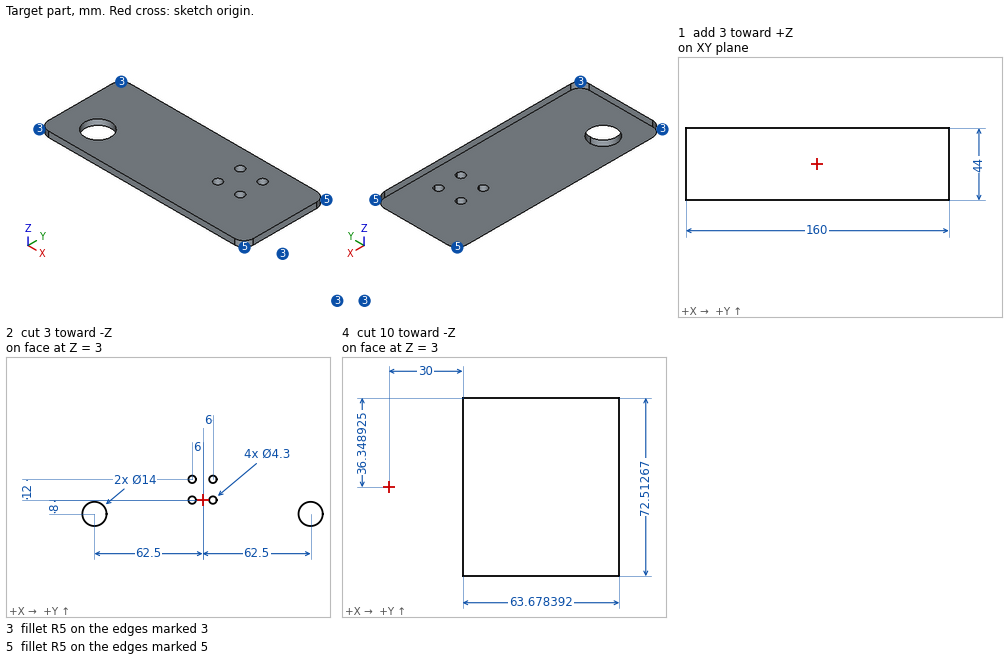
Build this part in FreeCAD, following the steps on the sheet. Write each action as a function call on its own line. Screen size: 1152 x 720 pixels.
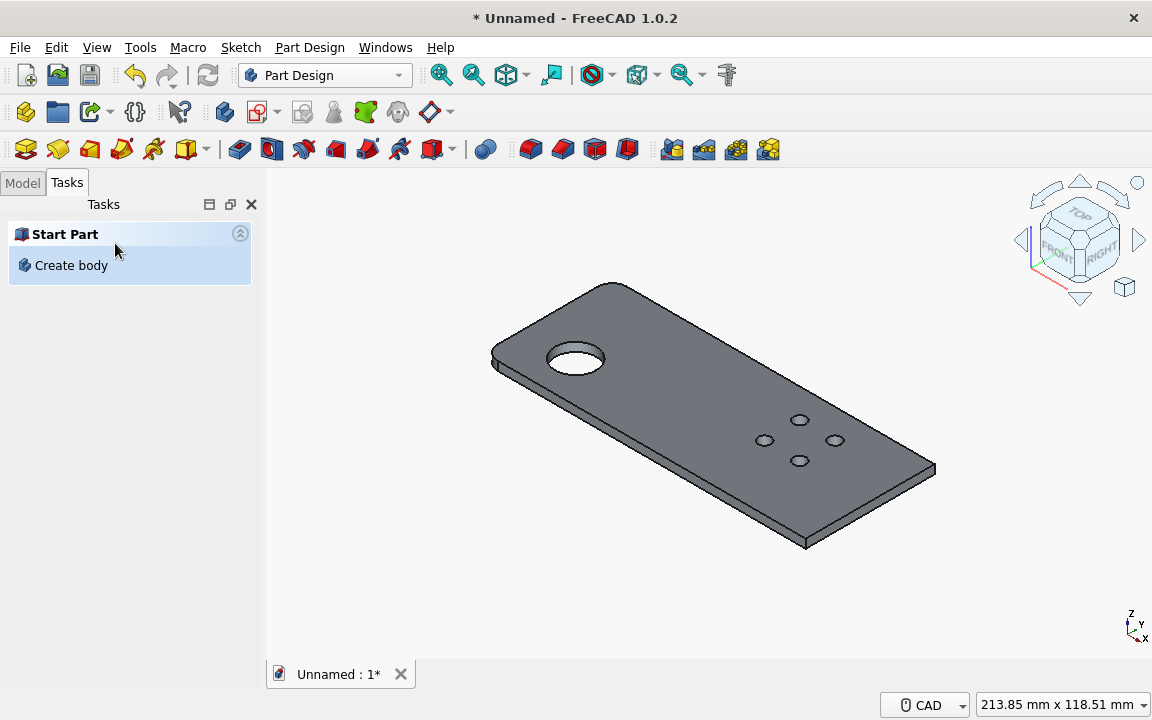
click(806, 544)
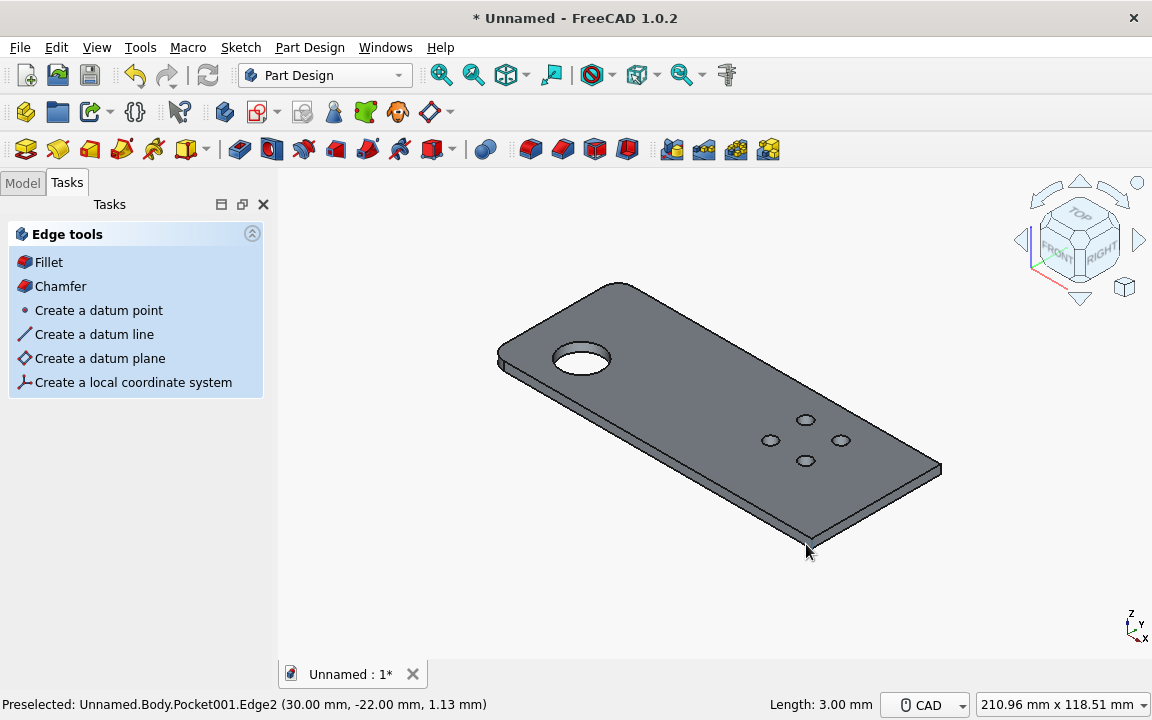
scroll(941, 468, up, 6)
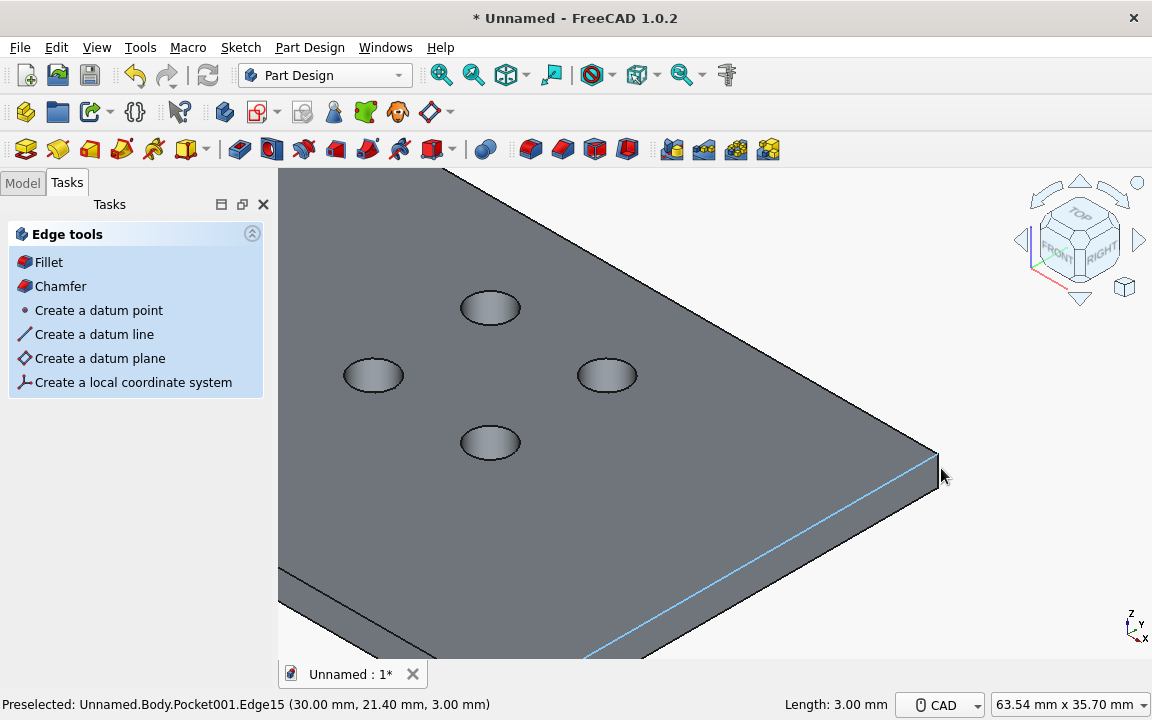
key(v)
key(f)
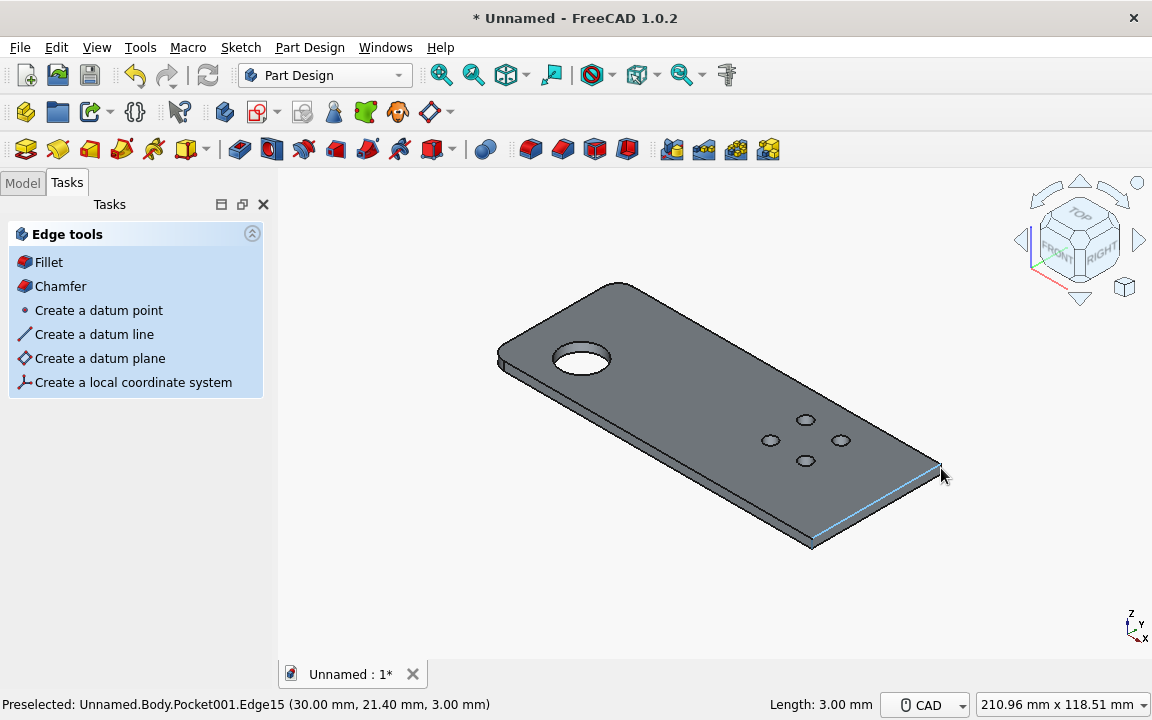
key(2)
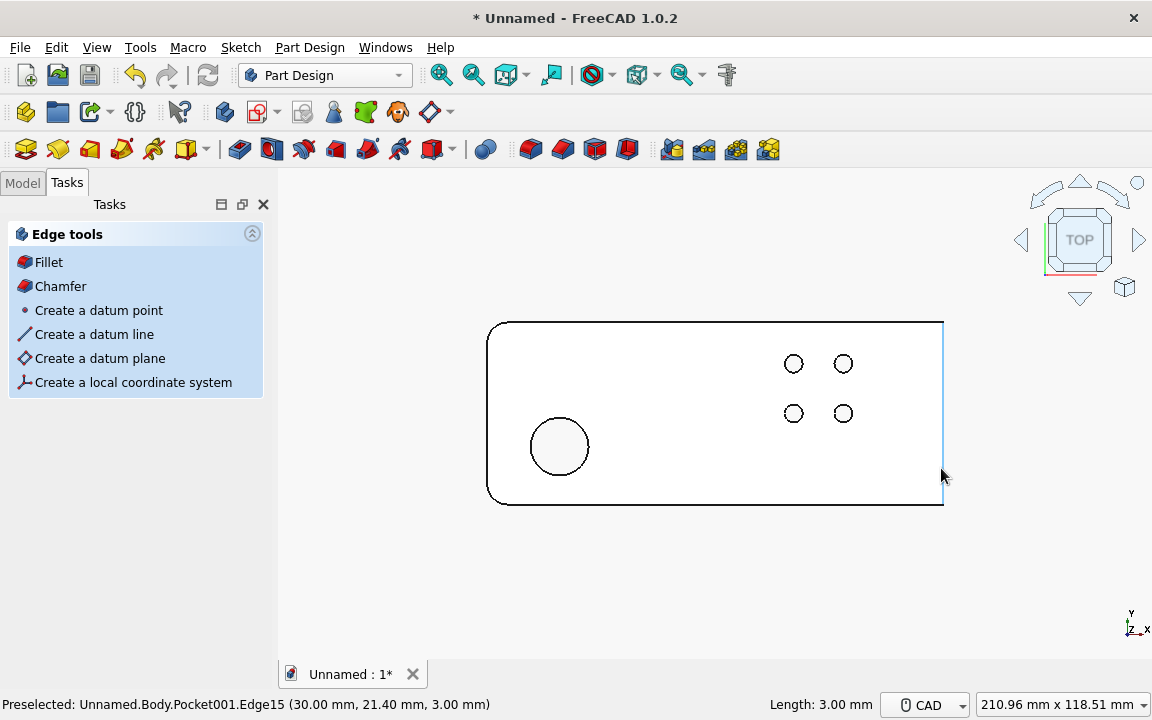
scroll(943, 321, up, 6)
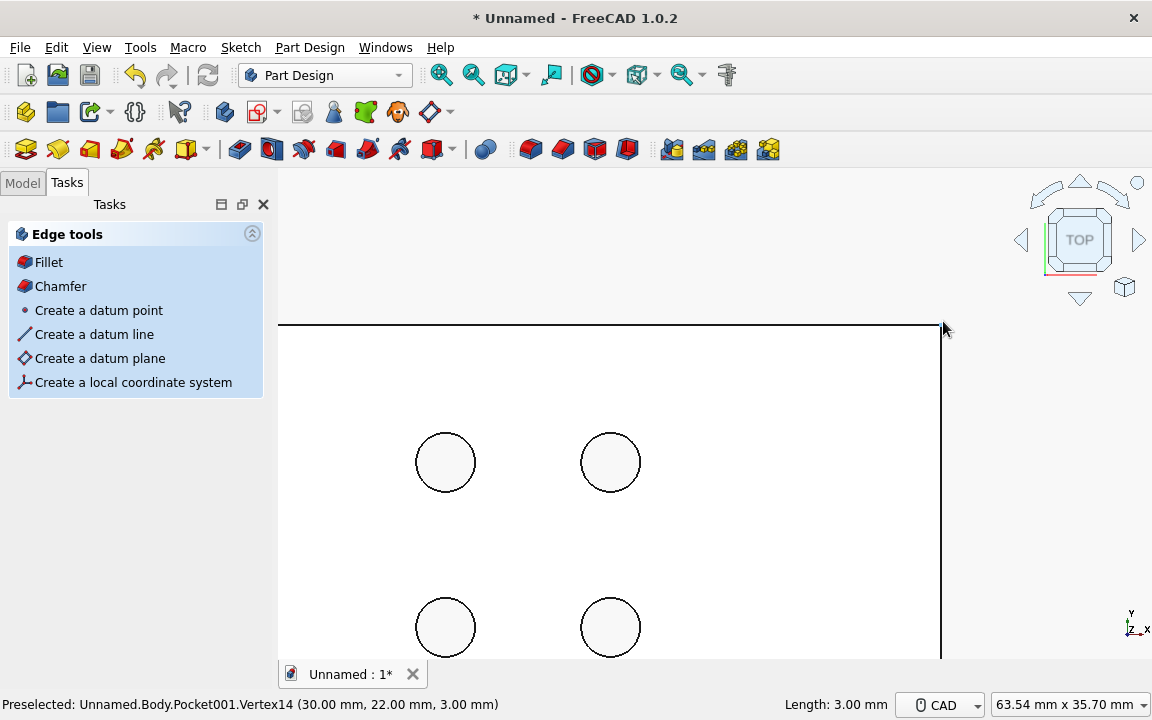
key(v)
key(f)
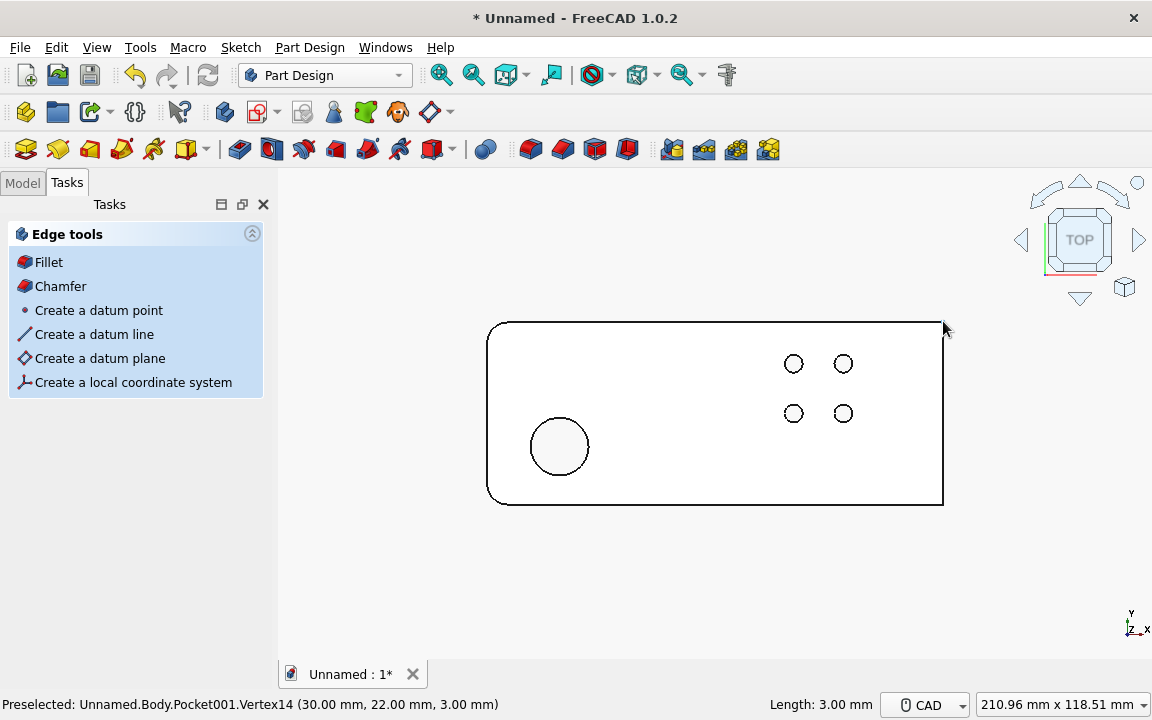
key(0)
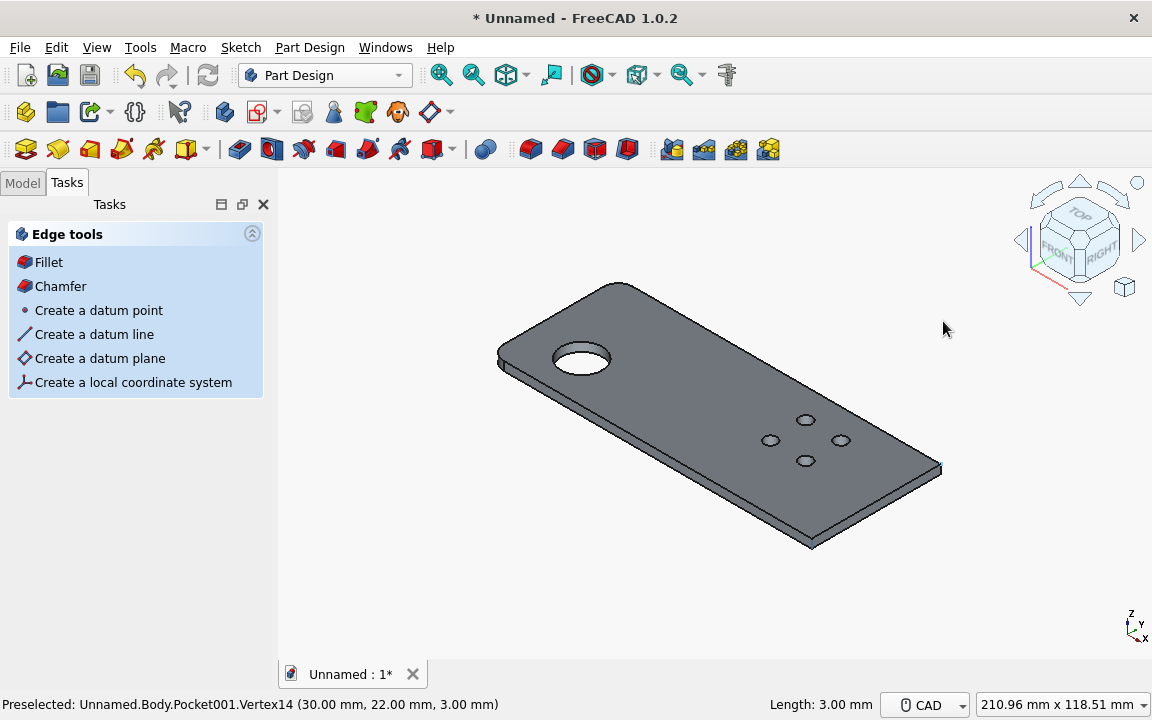
scroll(941, 468, up, 6)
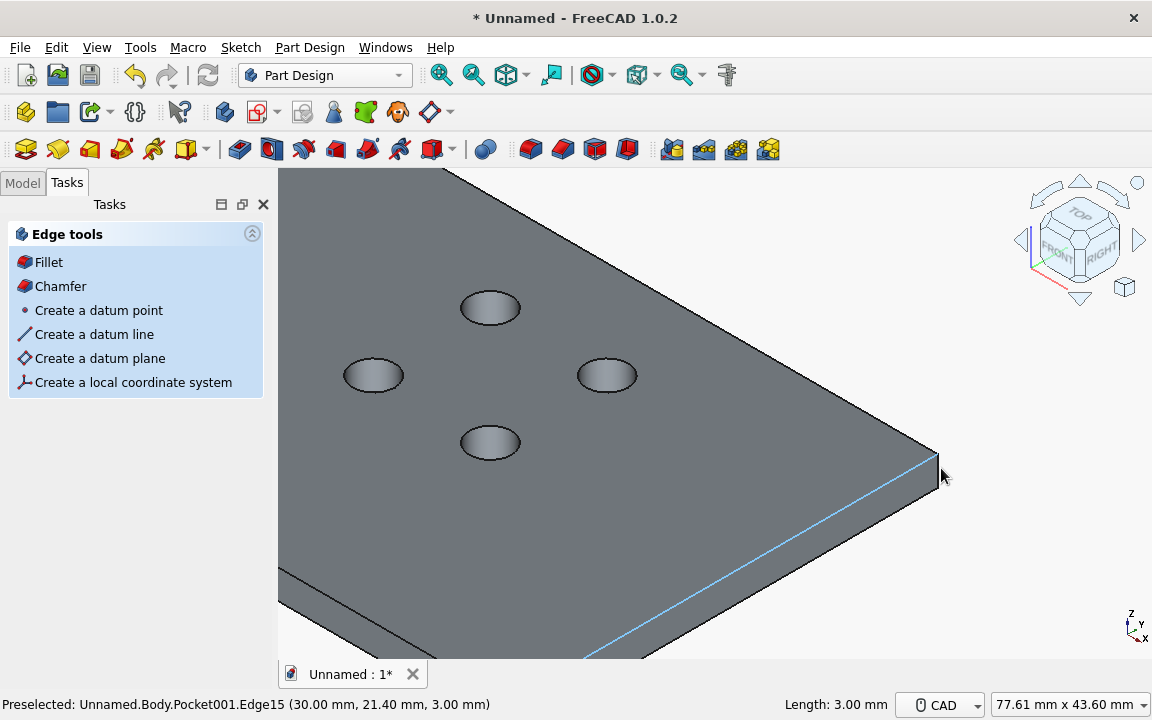
key(v)
key(f)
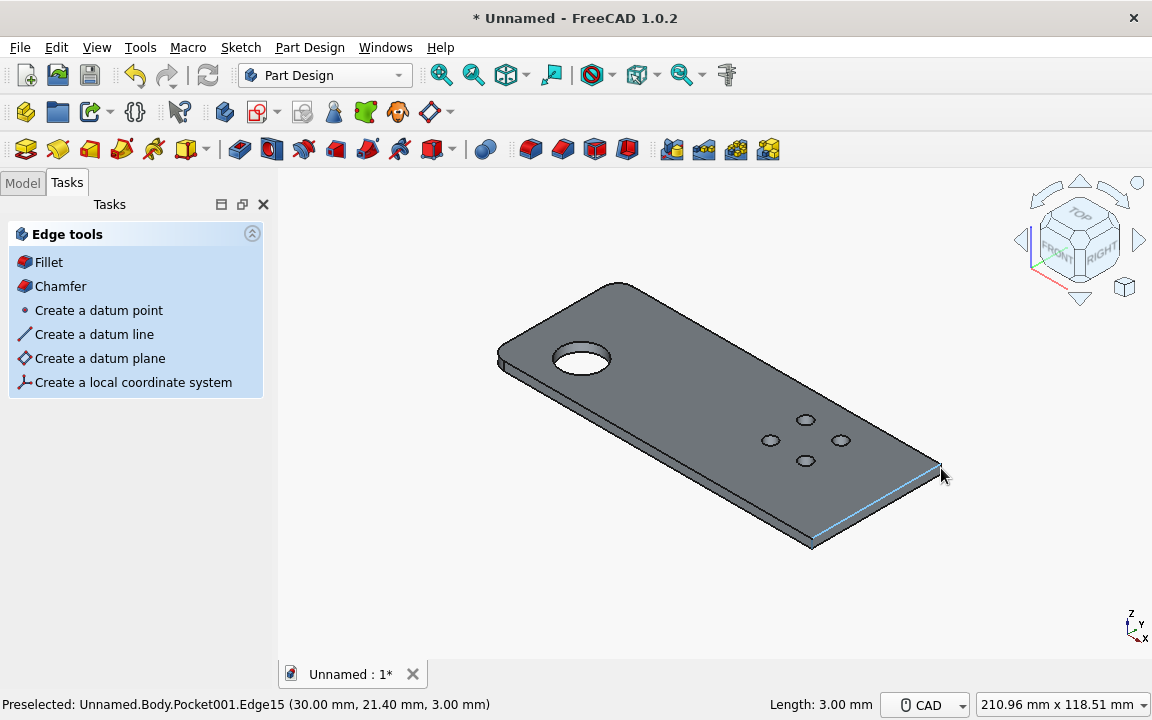
key(1)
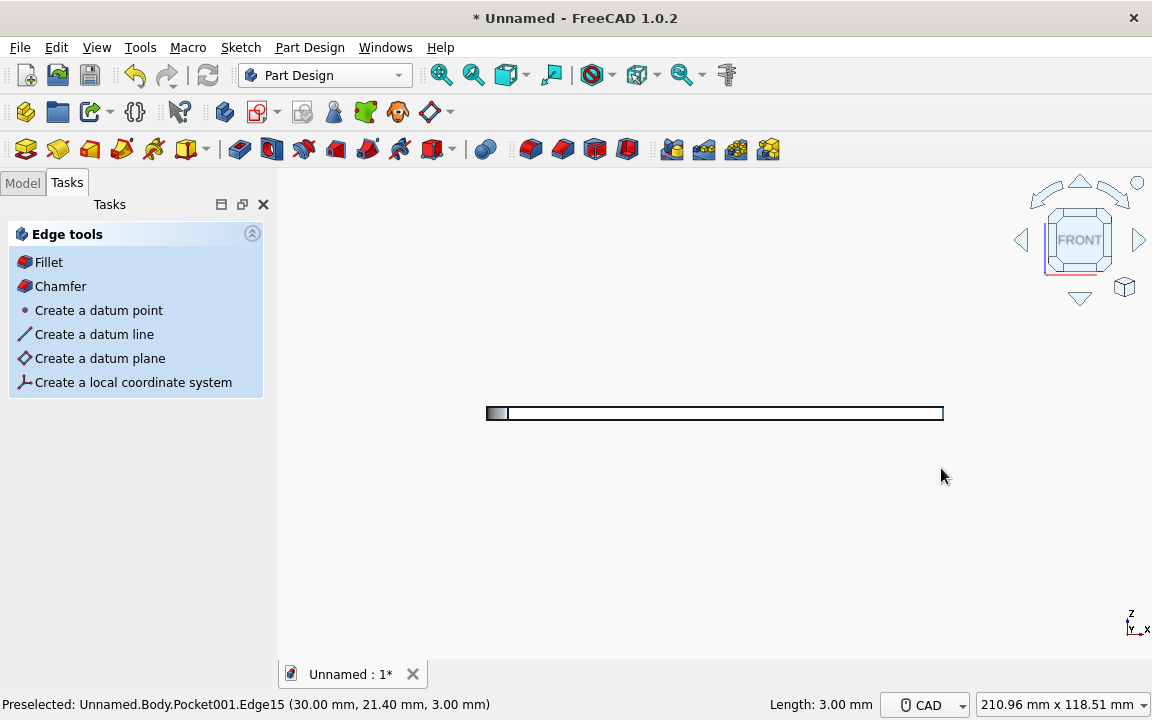
scroll(943, 413, up, 6)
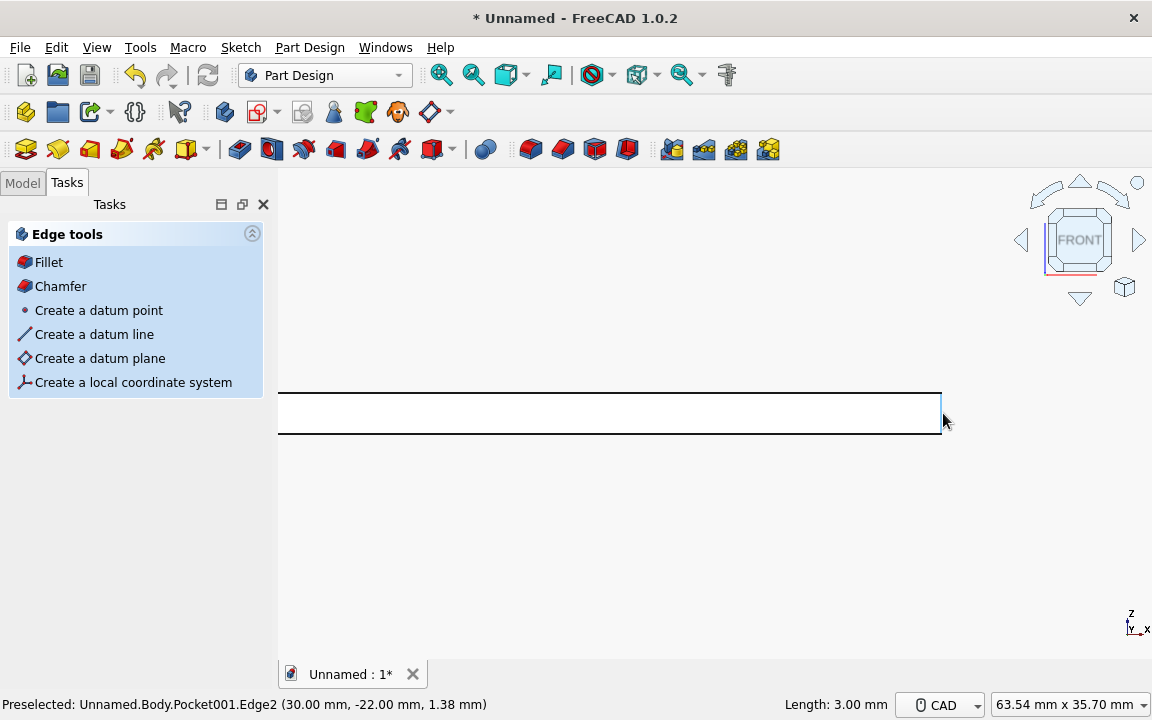
click(442, 76)